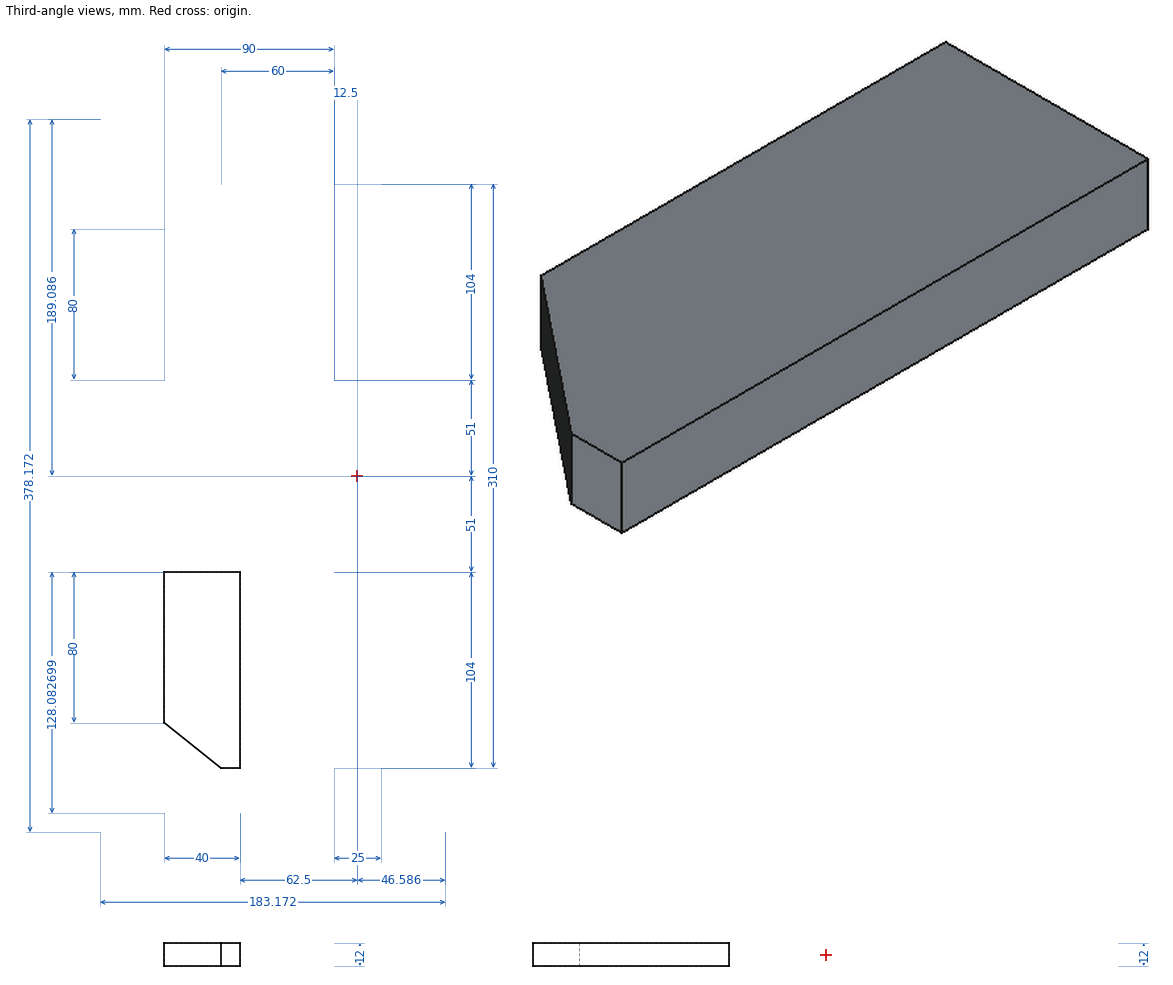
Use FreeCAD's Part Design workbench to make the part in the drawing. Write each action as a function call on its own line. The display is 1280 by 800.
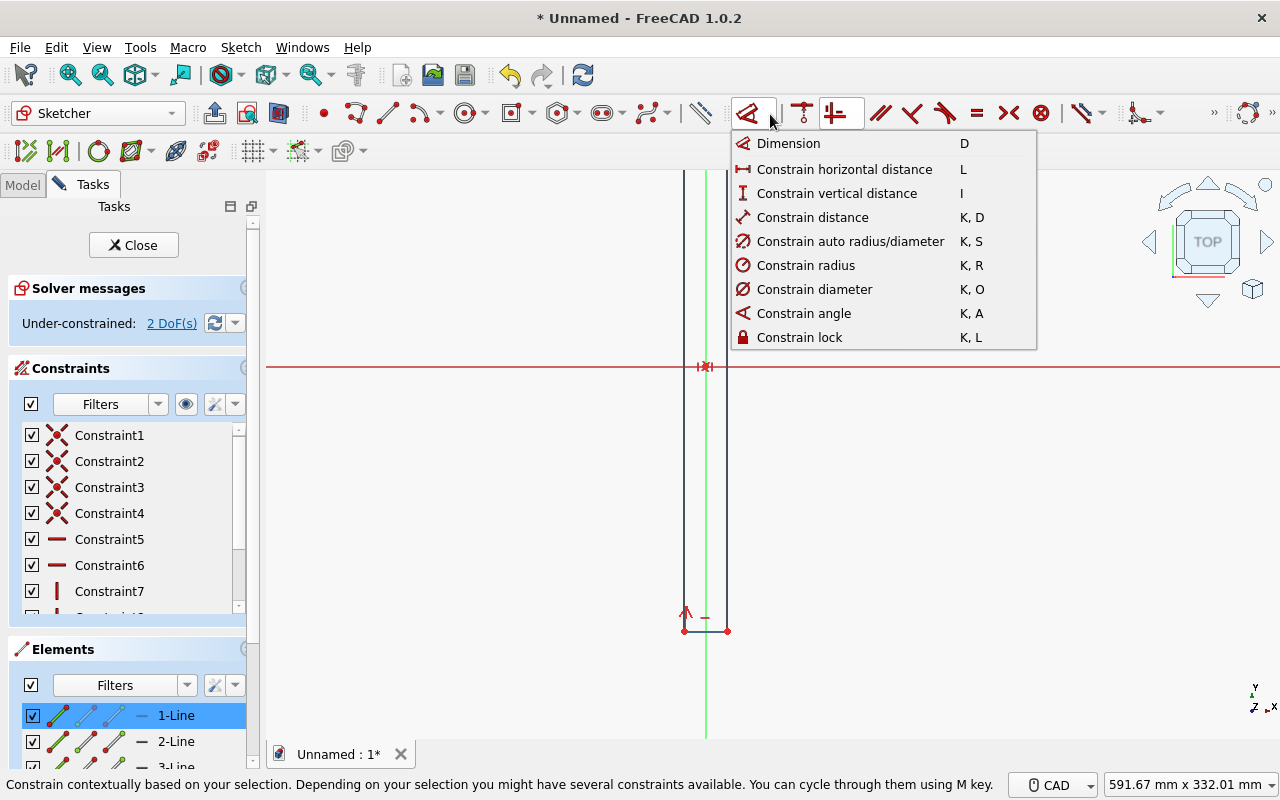
click(884, 169)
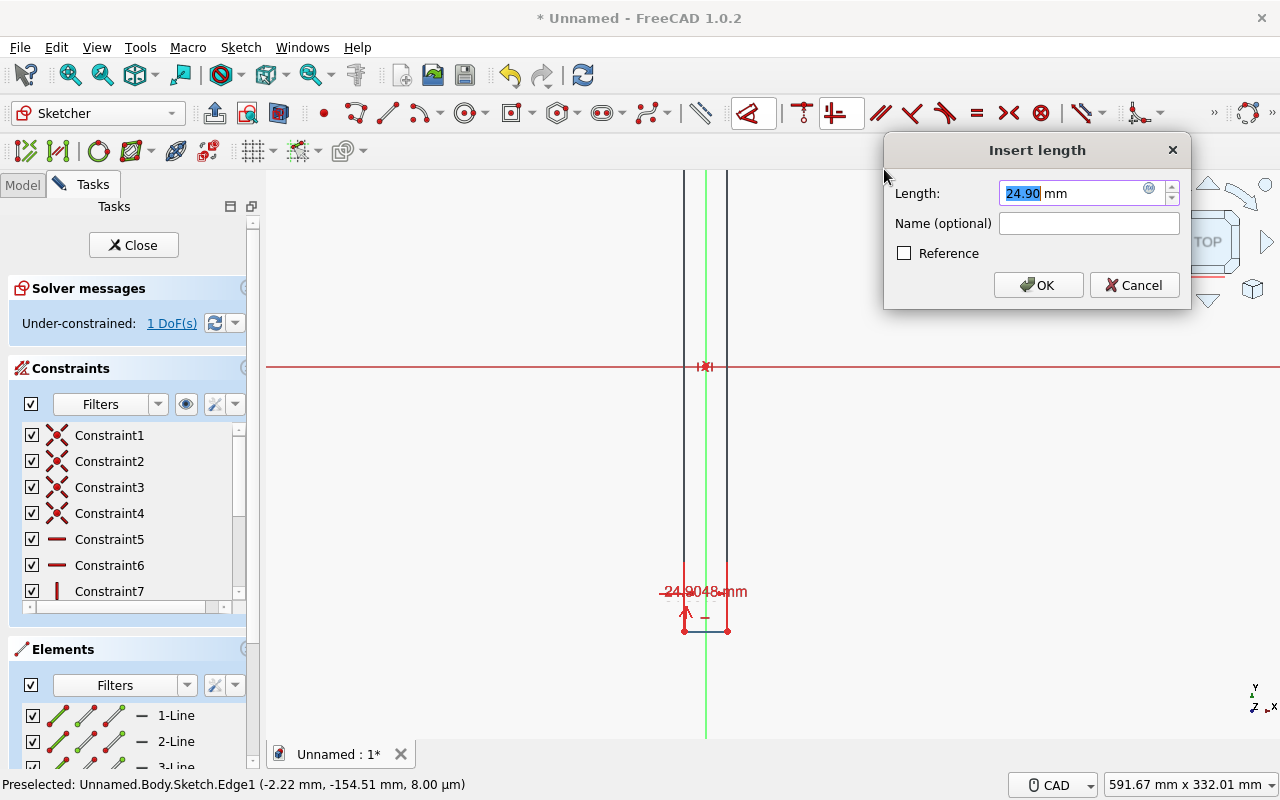
text(25)
key(Return)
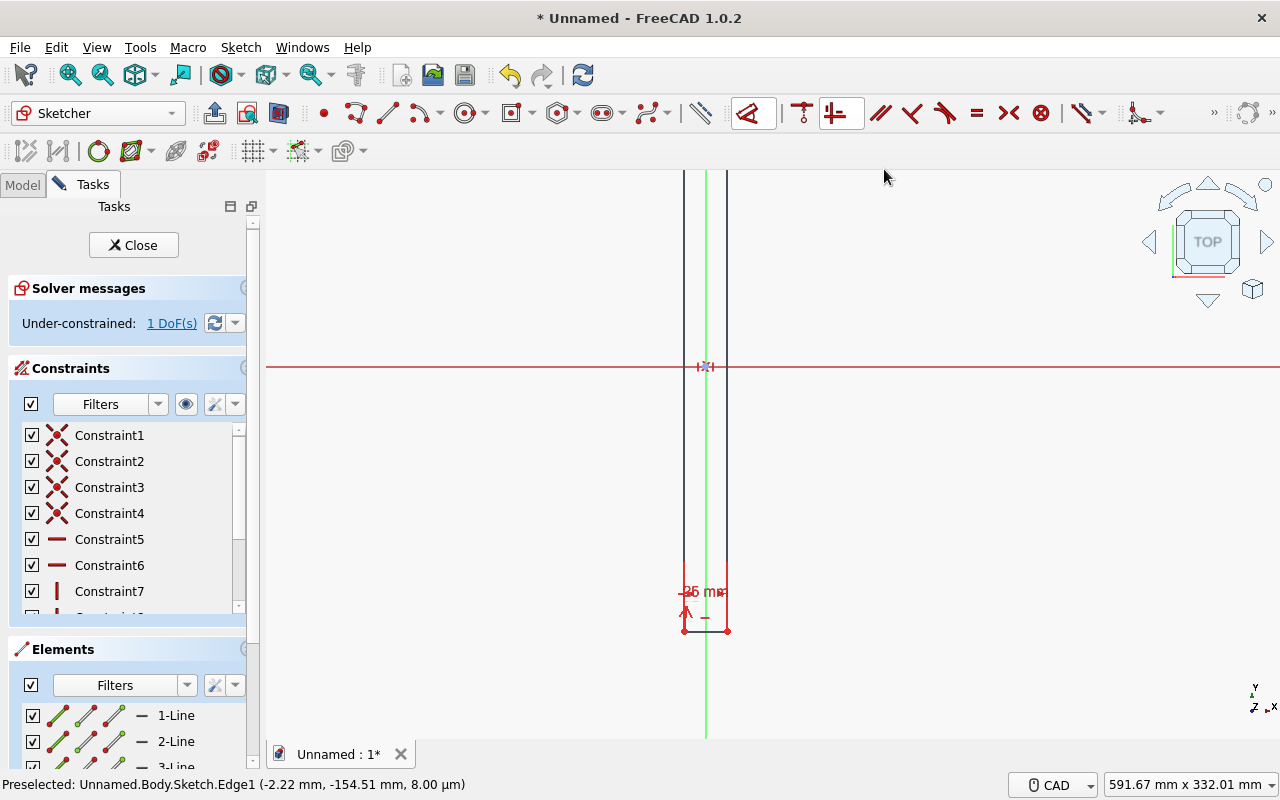
click(727, 473)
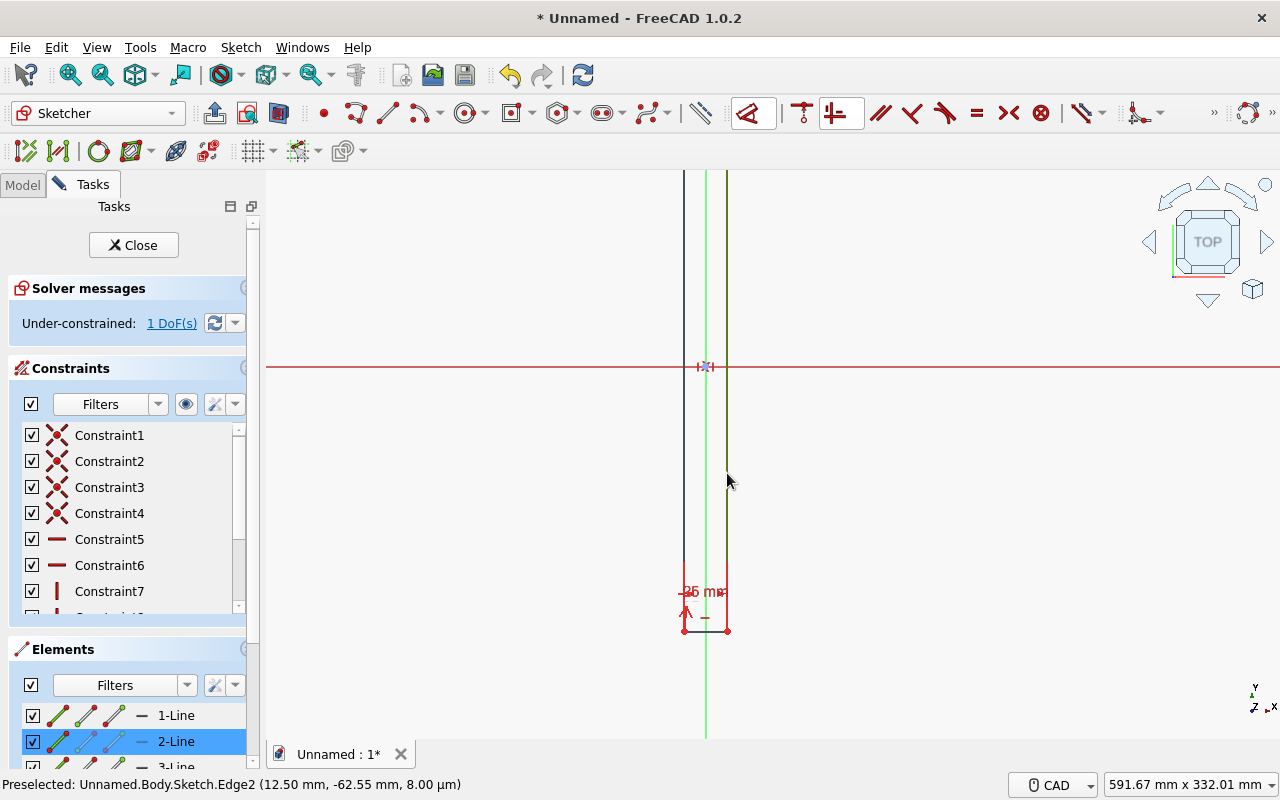
key(i)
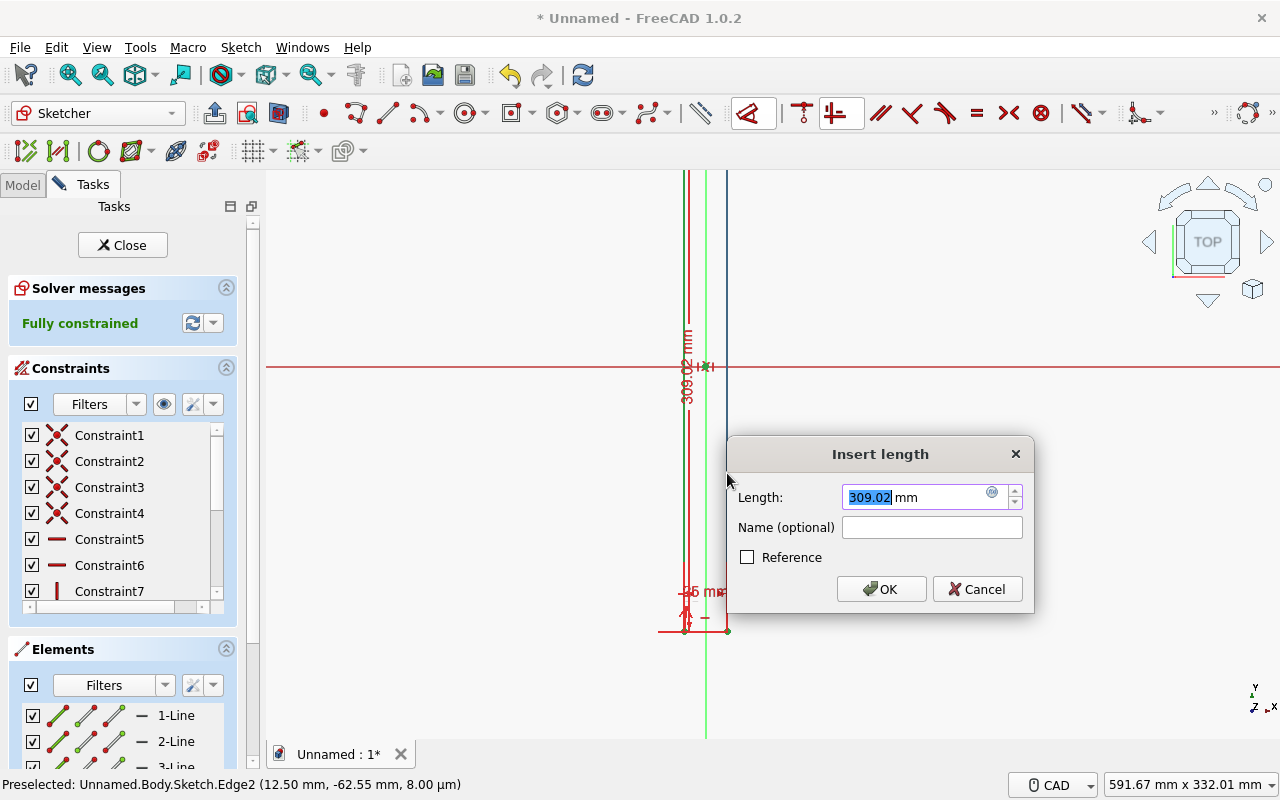
text(310)
key(Return)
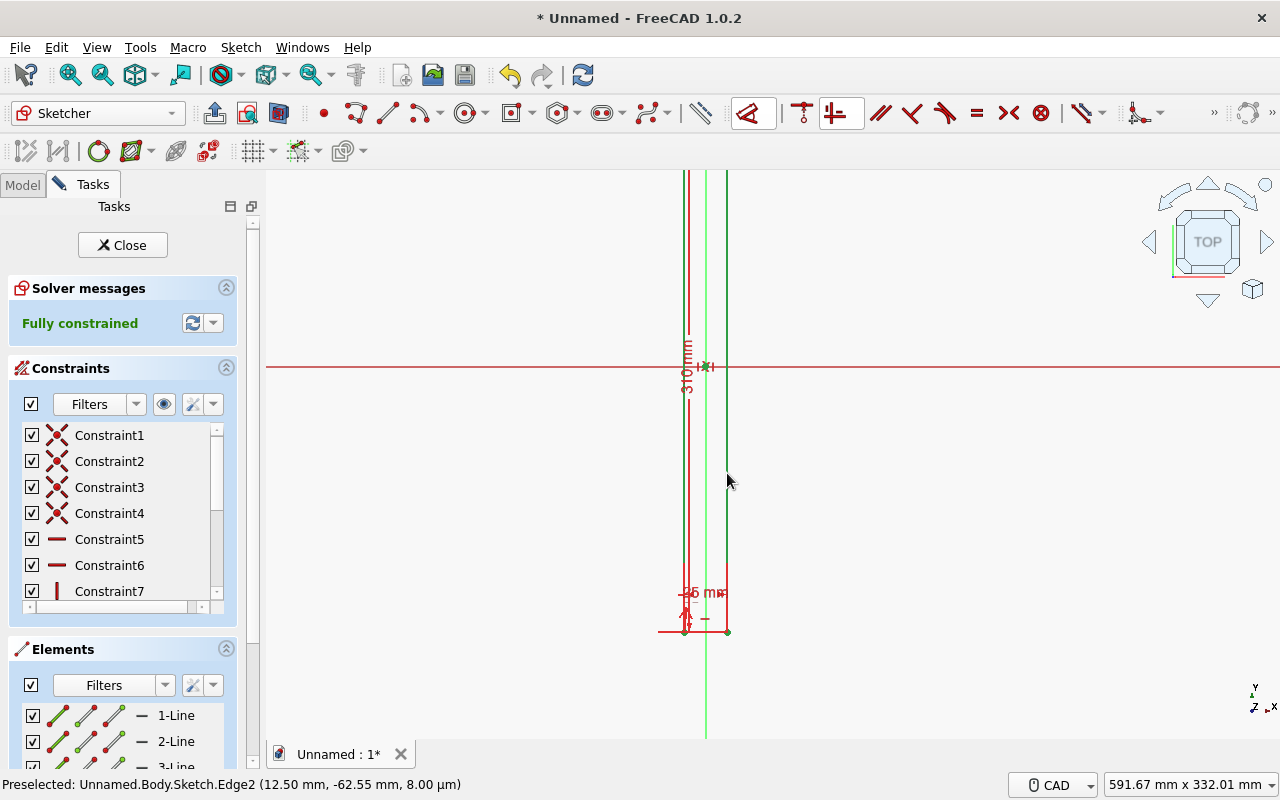
click(123, 245)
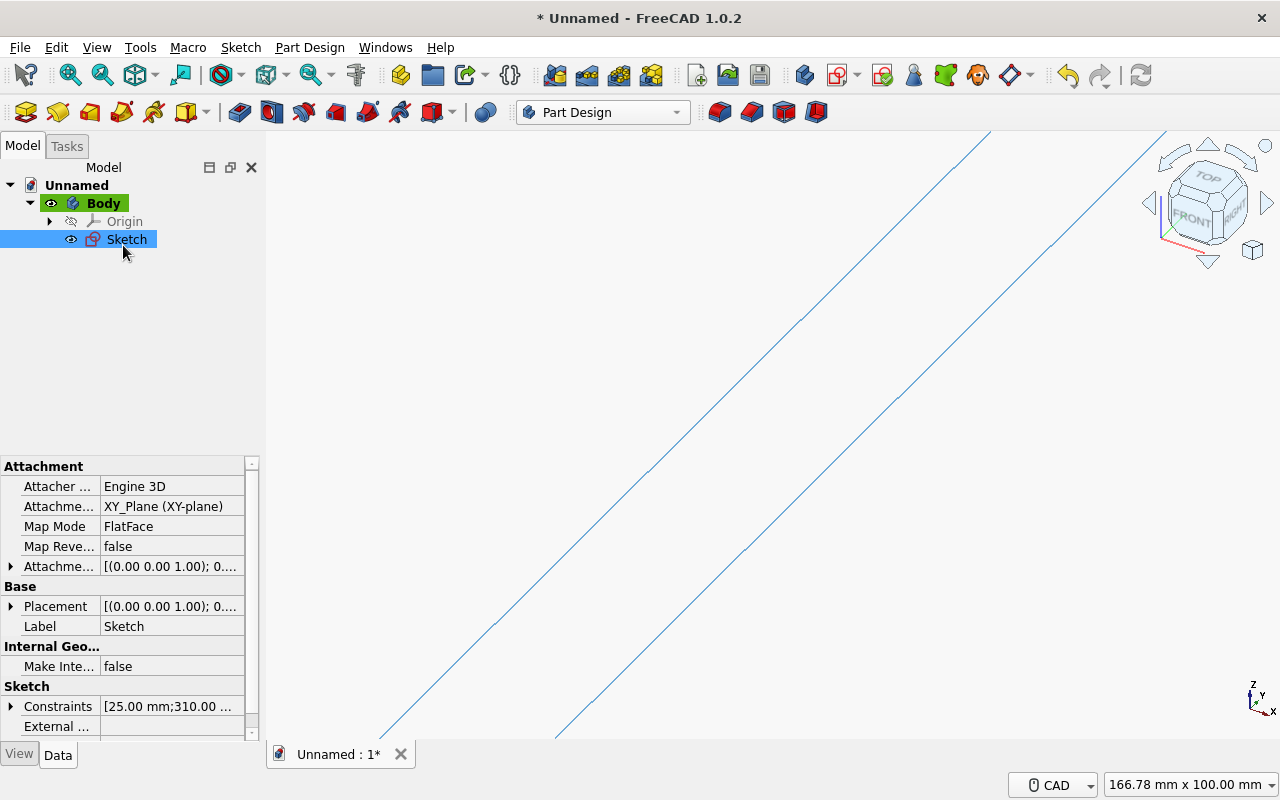
click(26, 112)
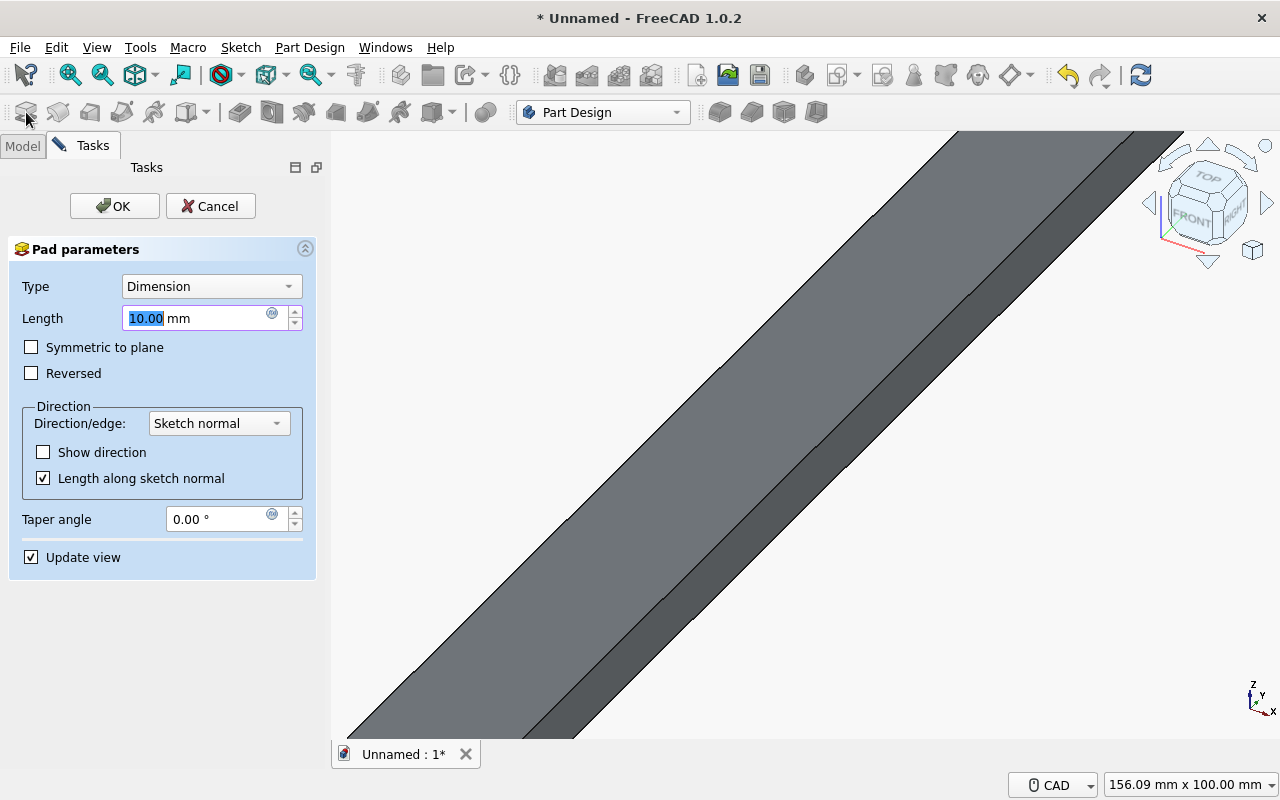
text(12)
key(Tab)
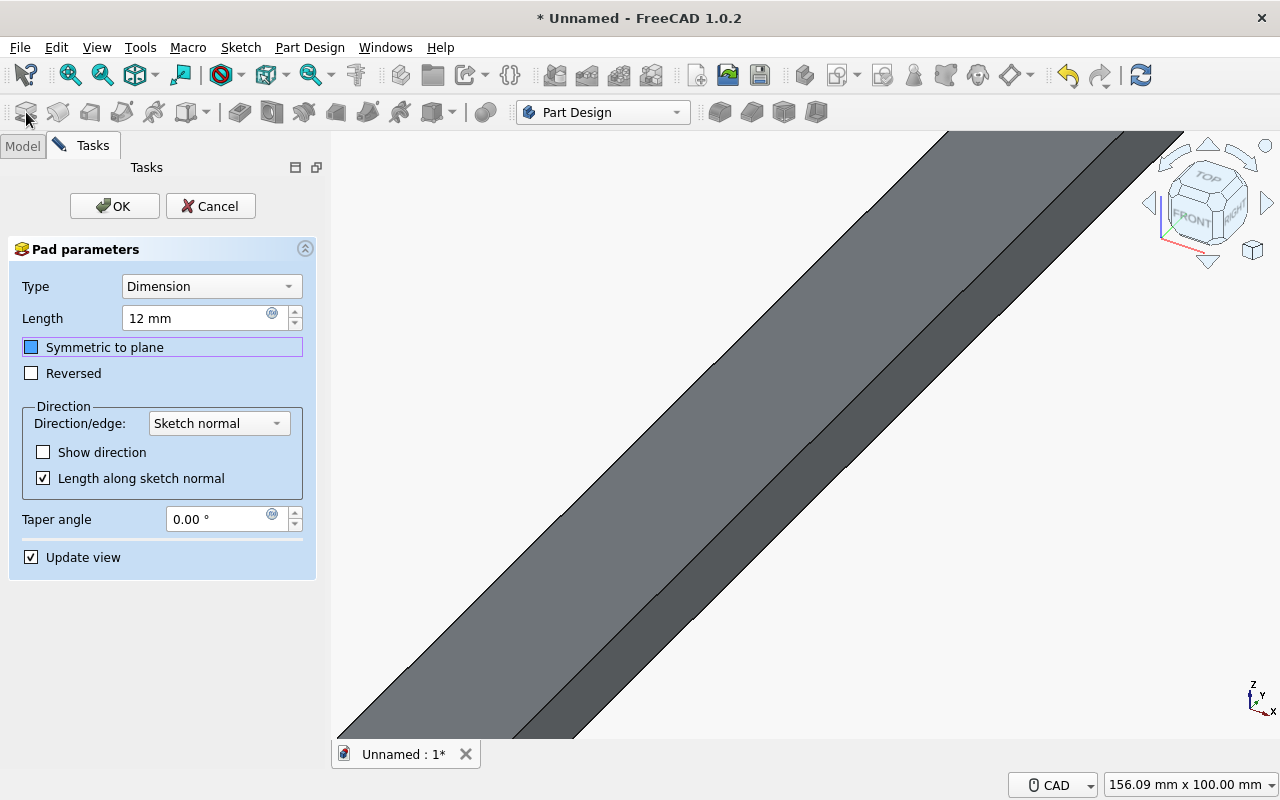
click(30, 347)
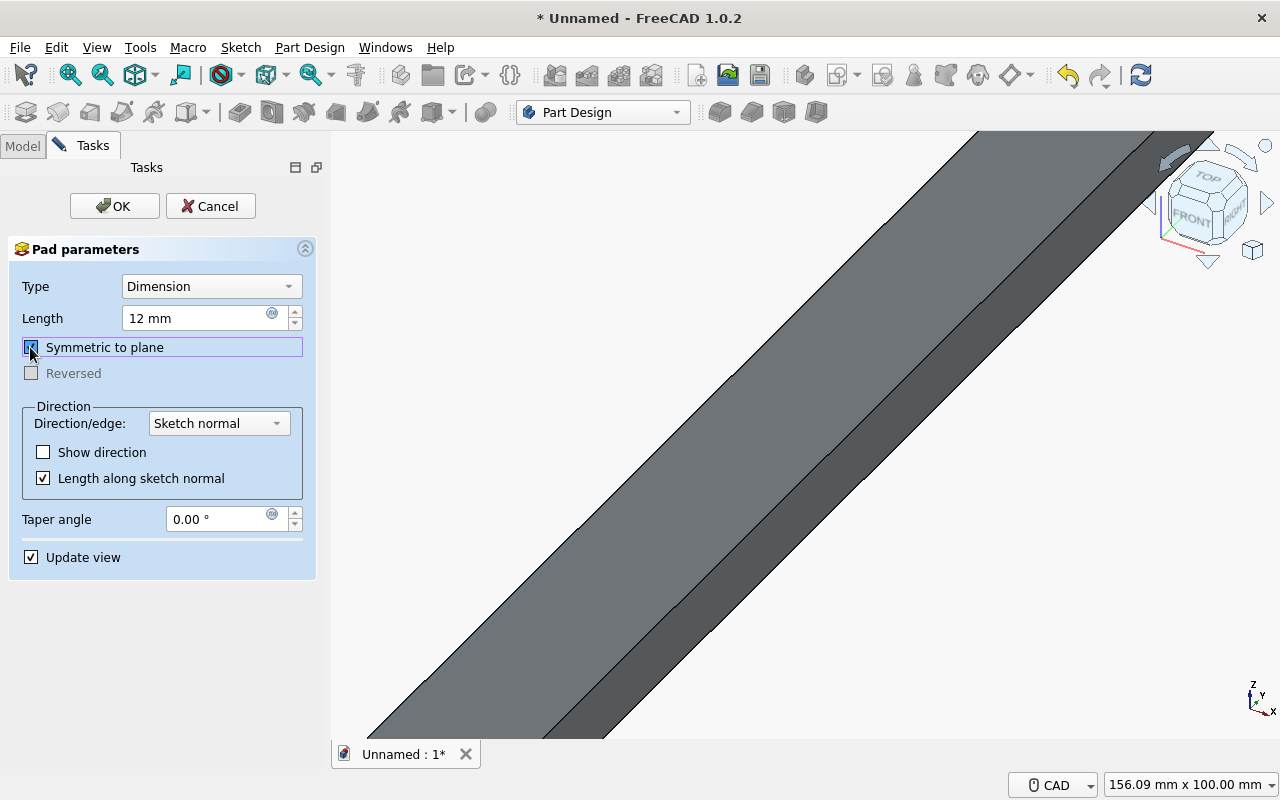
click(115, 206)